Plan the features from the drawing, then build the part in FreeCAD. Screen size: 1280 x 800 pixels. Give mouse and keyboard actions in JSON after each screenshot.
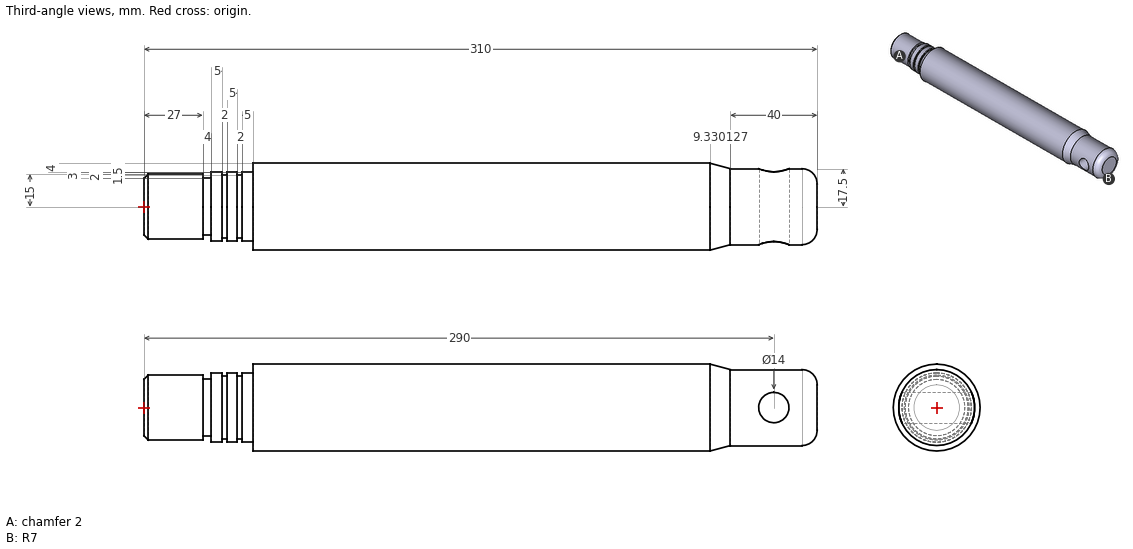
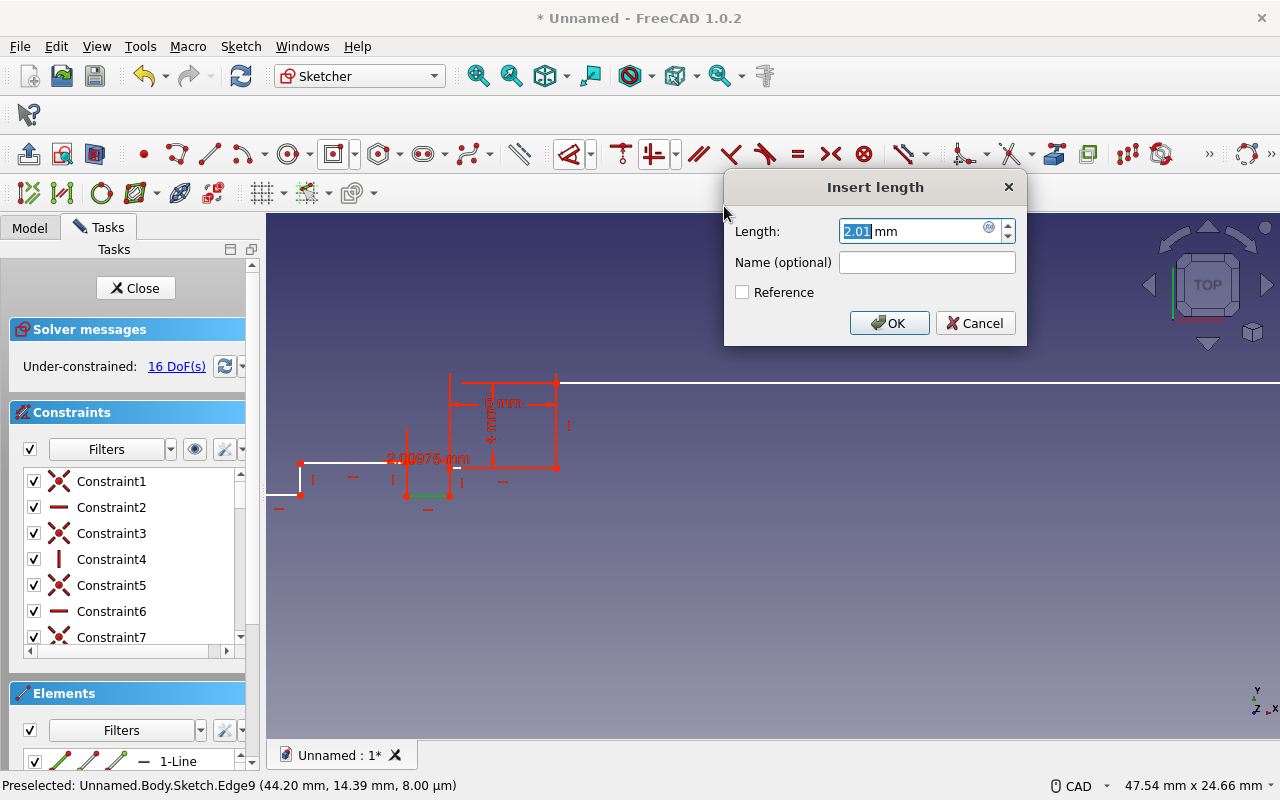
{"action": "type", "text": "2"}
{"action": "key", "text": "Return"}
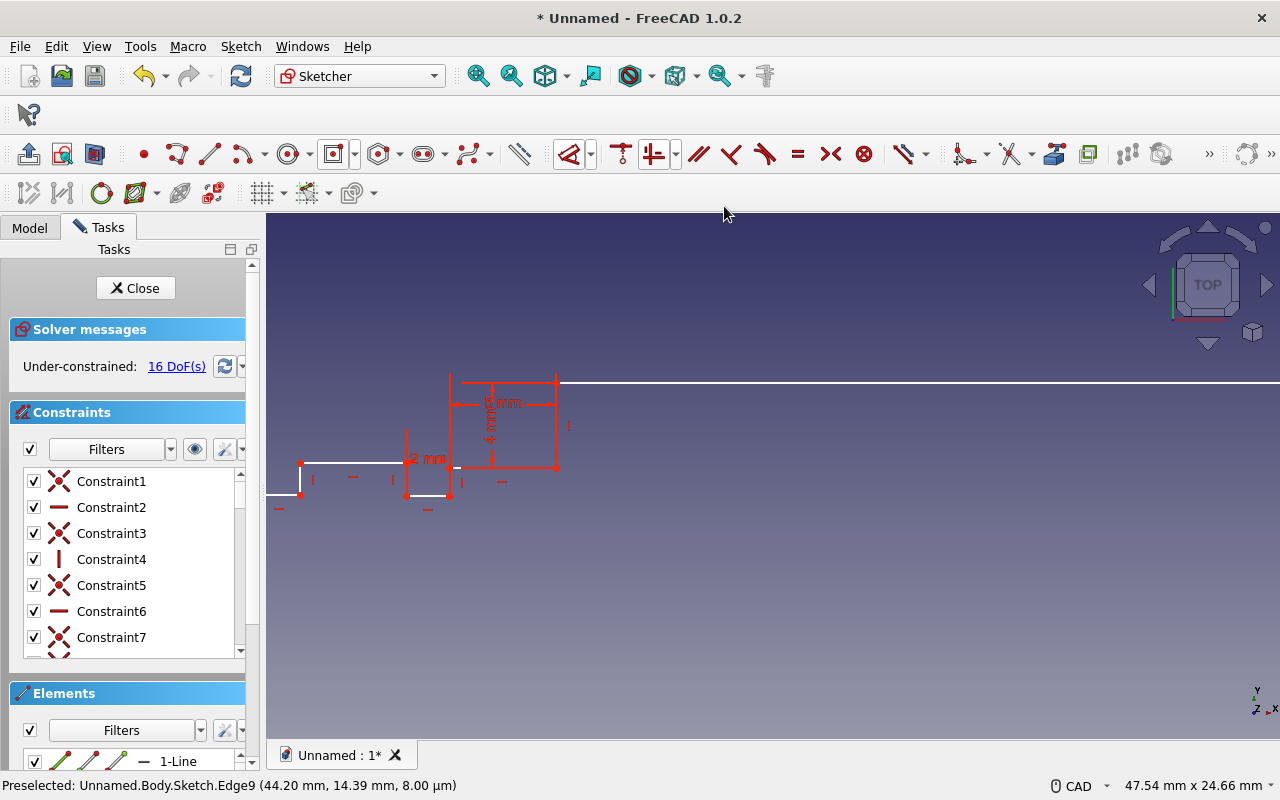
{"action": "left_click", "coordinate": [375, 463]}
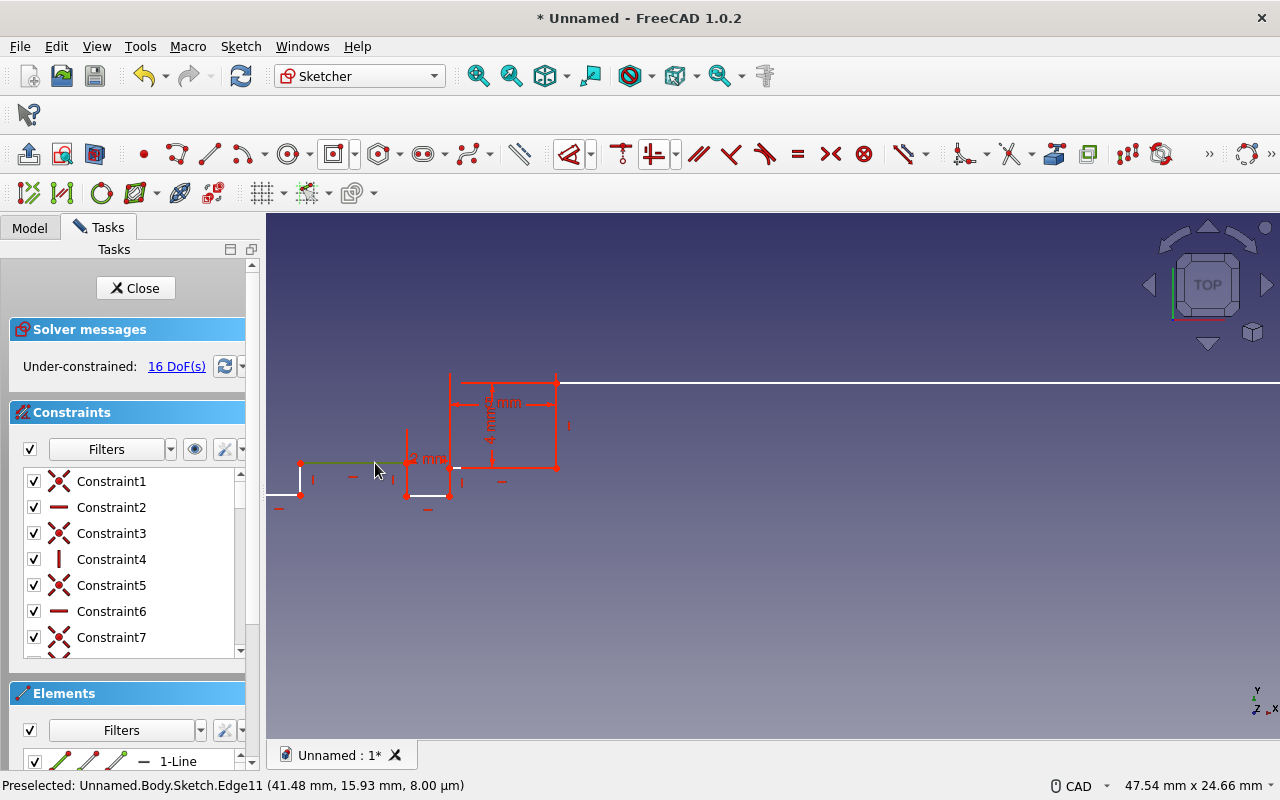
{"action": "left_click", "coordinate": [590, 154]}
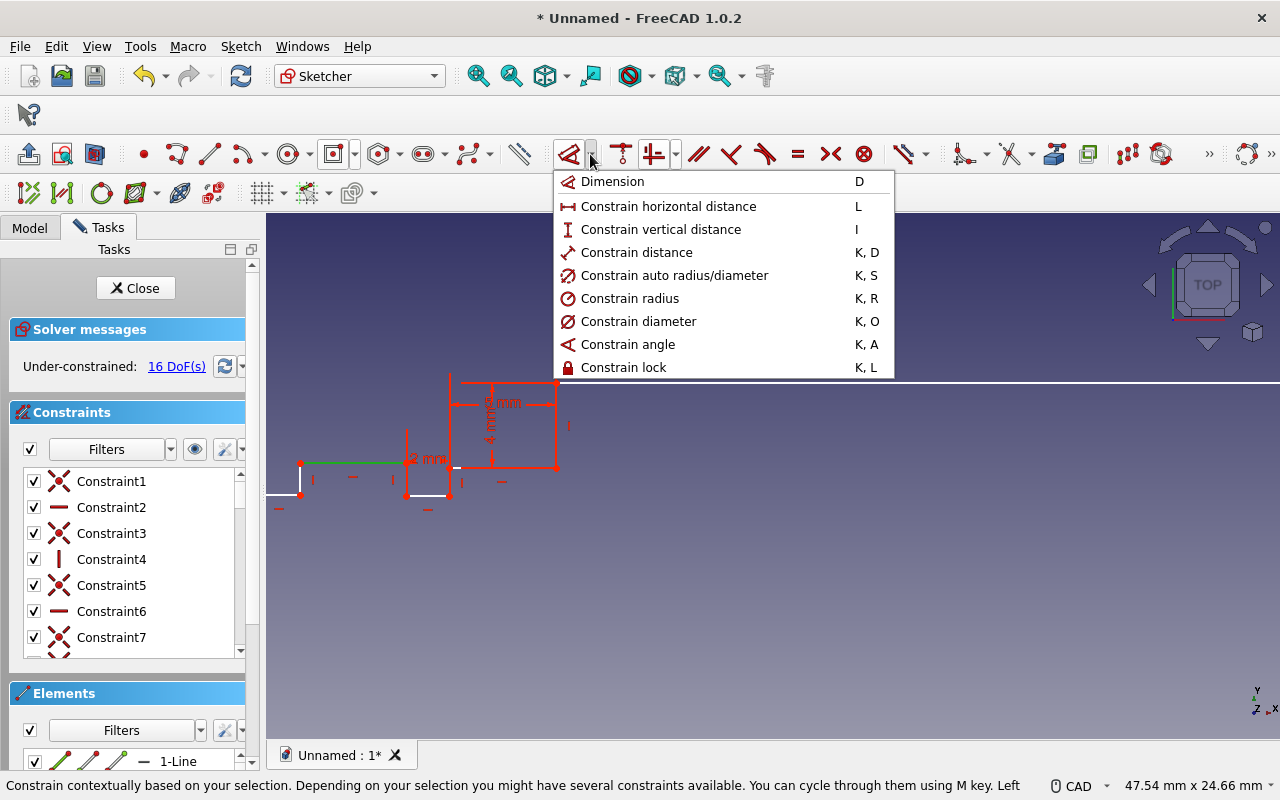
{"action": "left_click", "coordinate": [724, 206]}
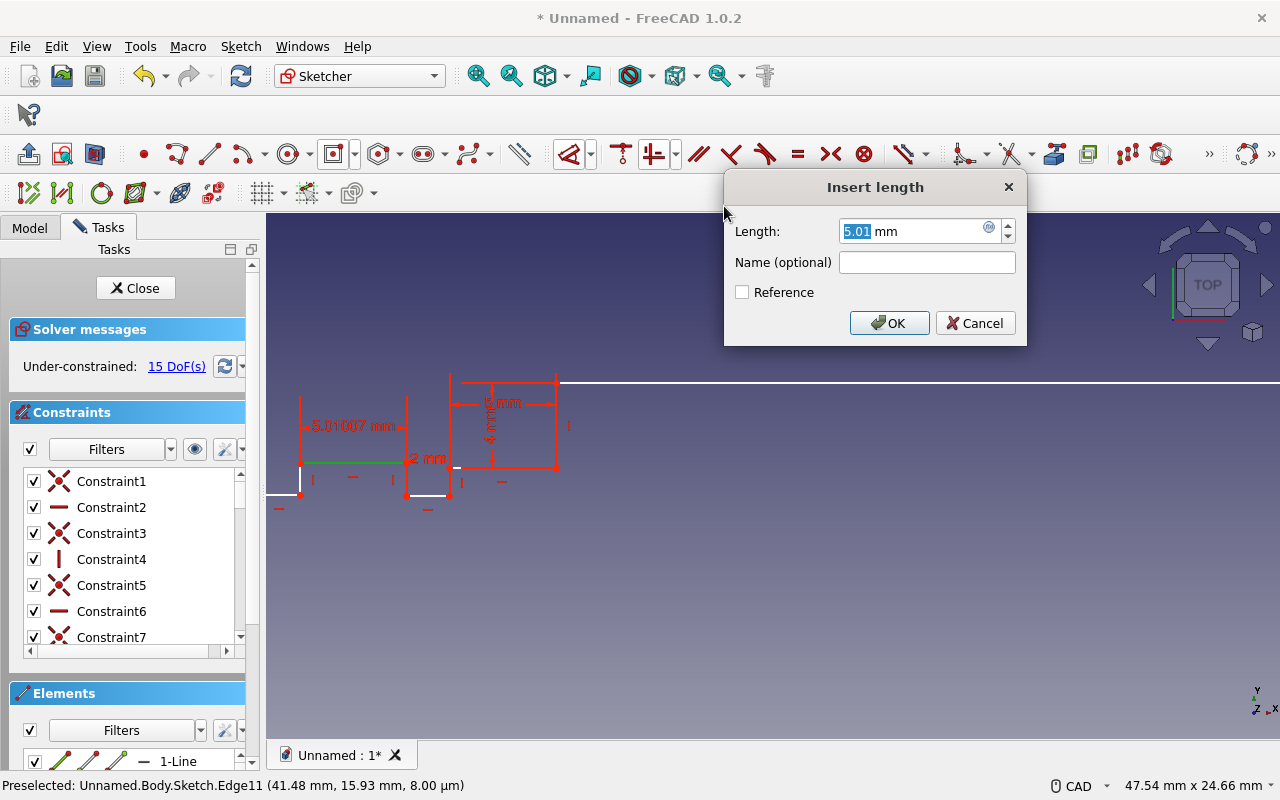
{"action": "type", "text": "5"}
{"action": "key", "text": "Return"}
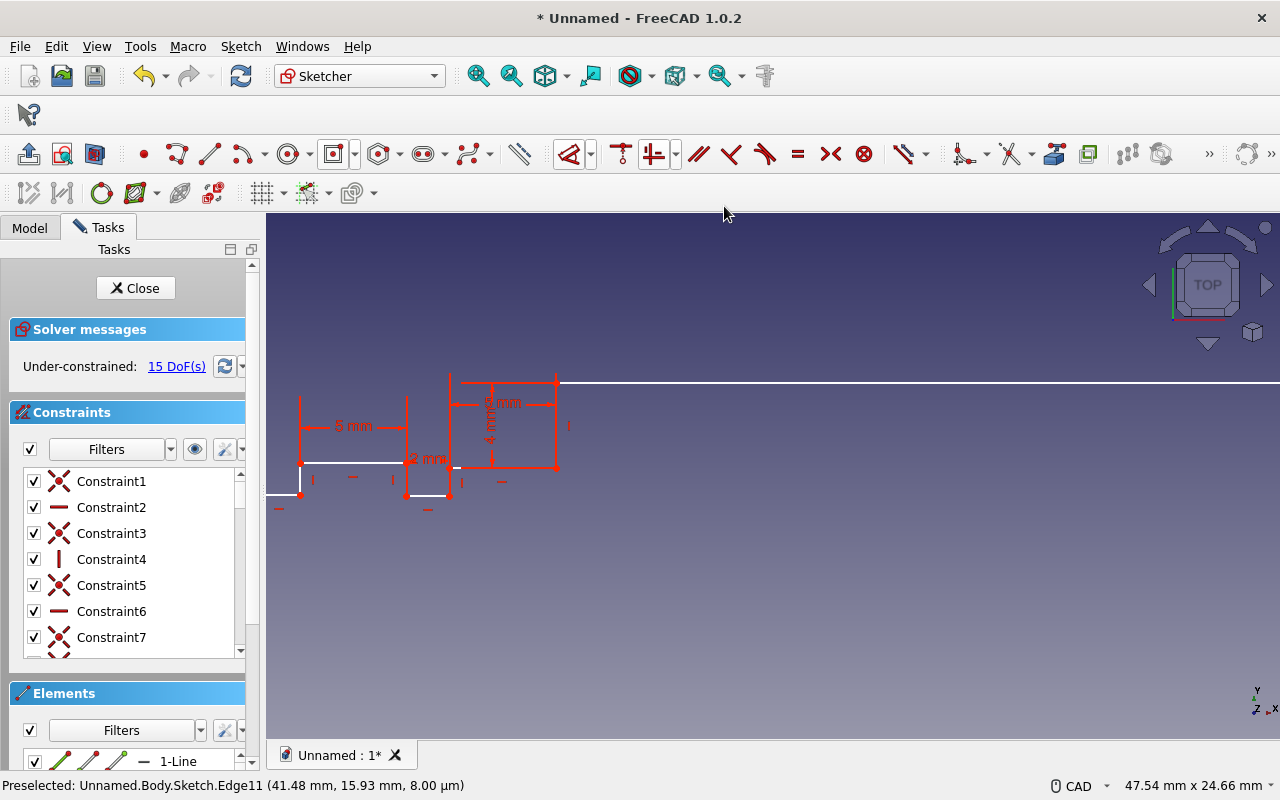
{"action": "scroll", "coordinate": [496, 465], "scroll_direction": "down", "scroll_amount": 12}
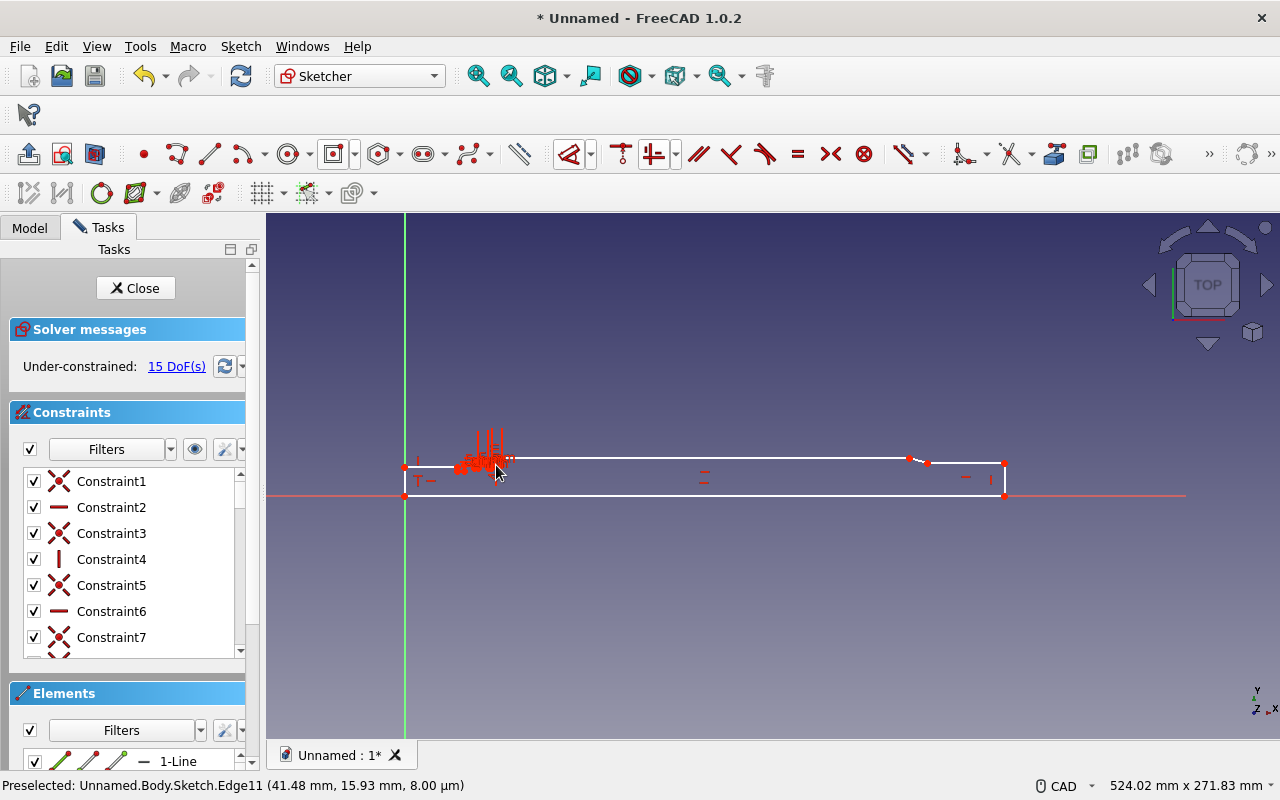
{"action": "scroll", "coordinate": [477, 468], "scroll_direction": "up", "scroll_amount": 13}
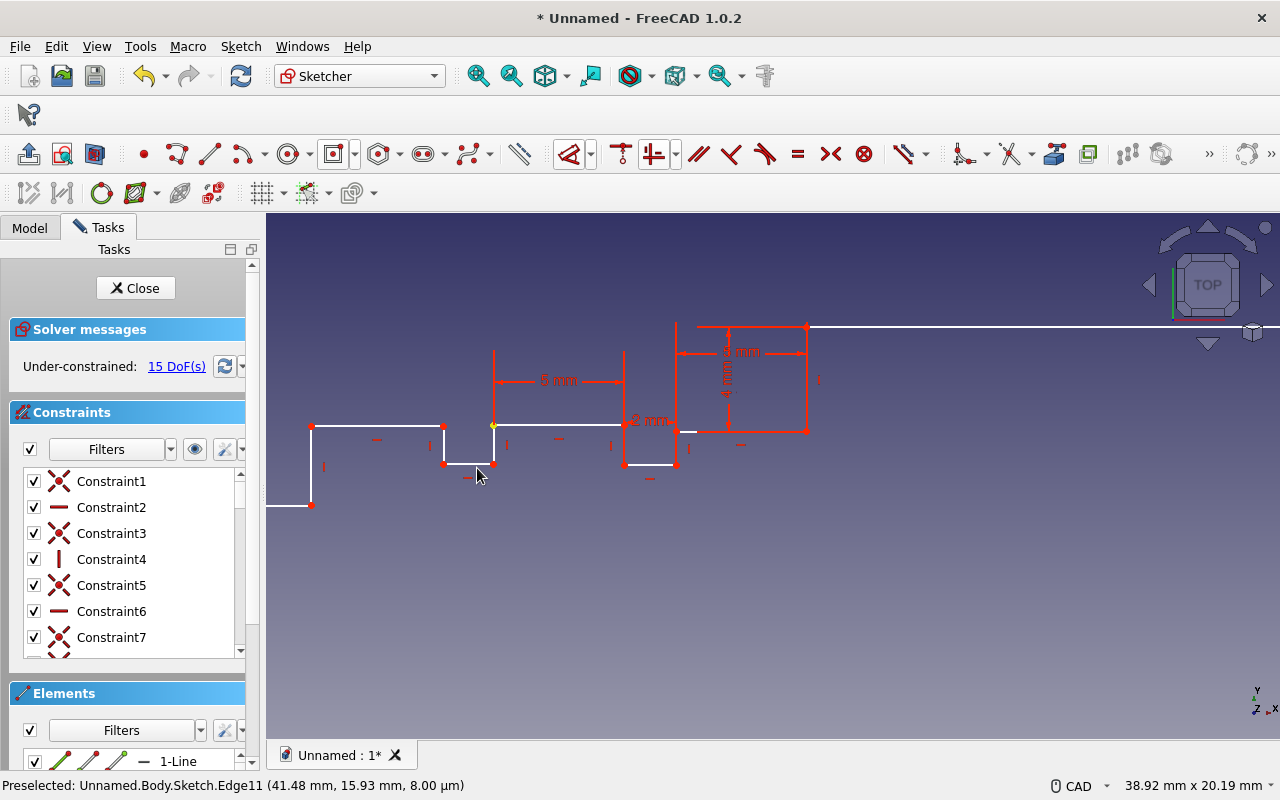
{"action": "left_click", "coordinate": [479, 464]}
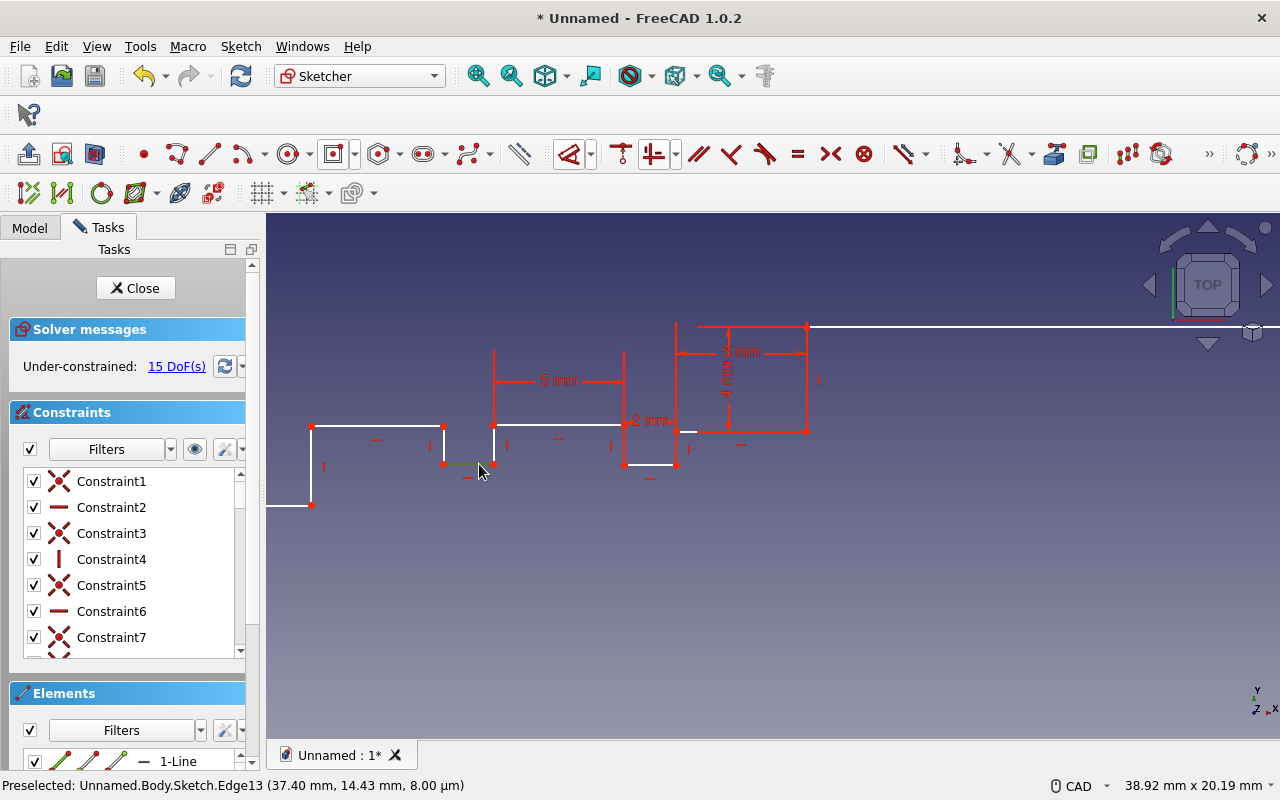
{"action": "left_click", "coordinate": [590, 154]}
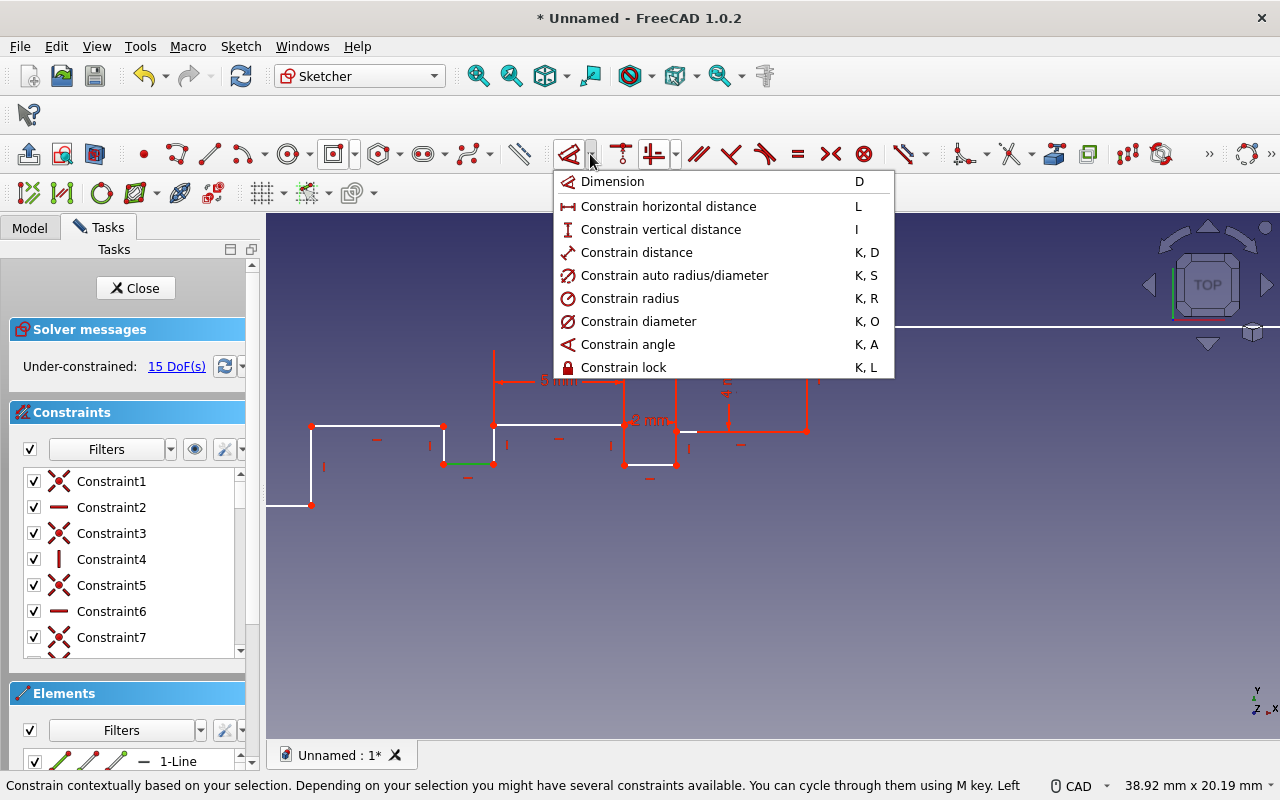
{"action": "left_click", "coordinate": [724, 206]}